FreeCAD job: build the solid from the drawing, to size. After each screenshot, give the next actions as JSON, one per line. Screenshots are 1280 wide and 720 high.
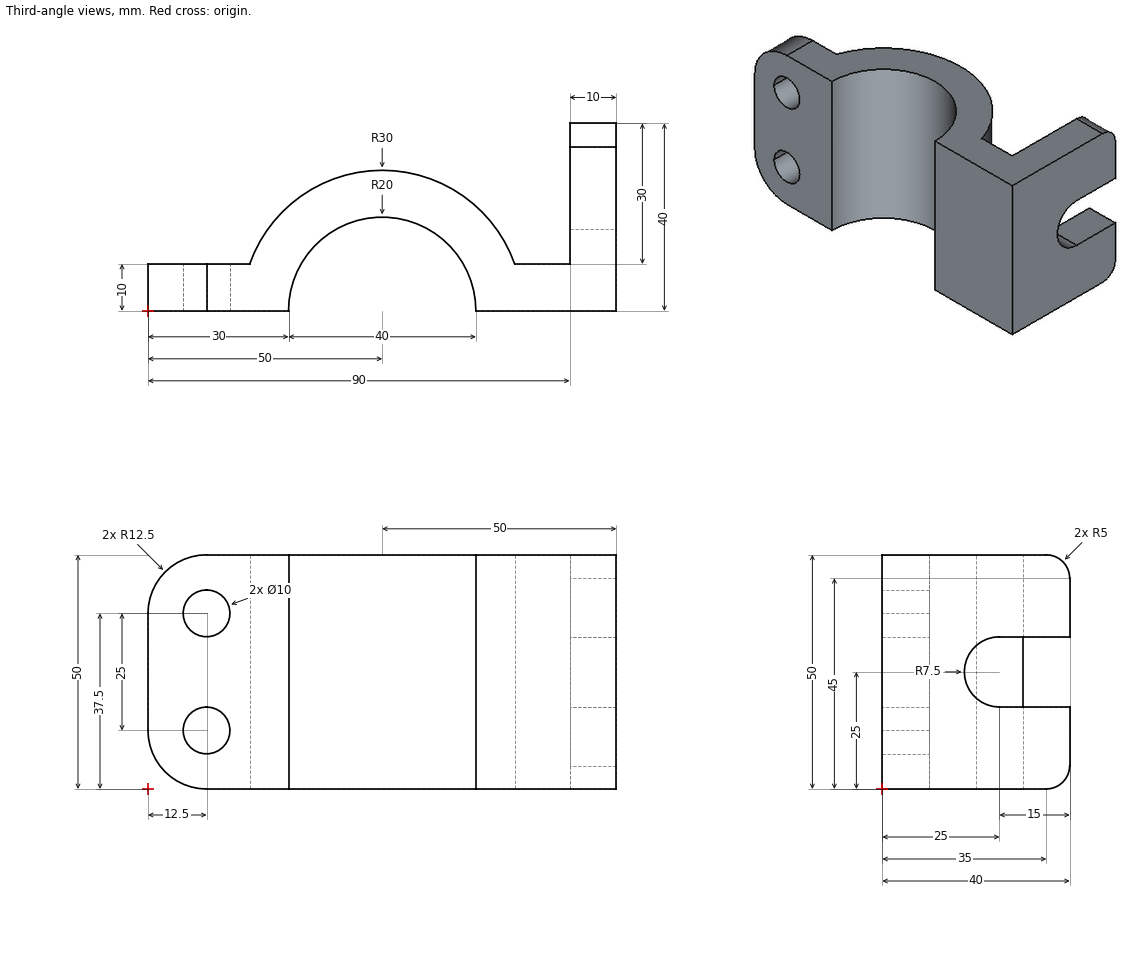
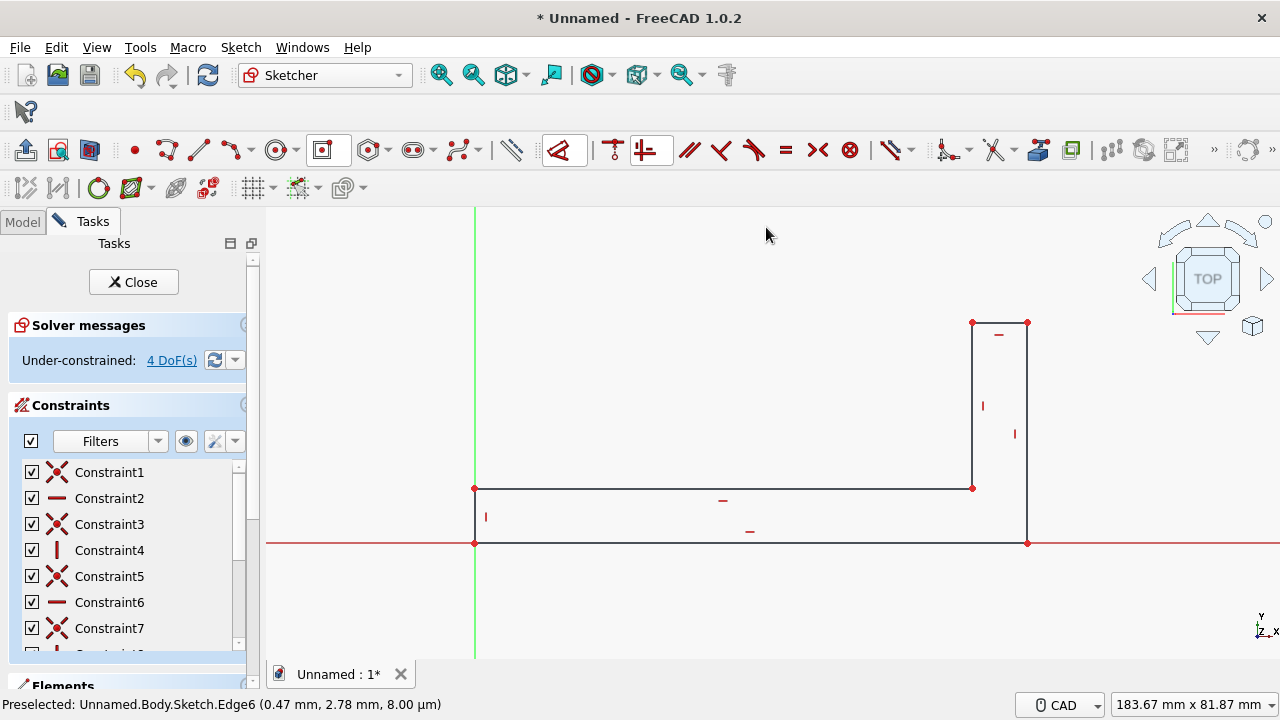
{"action": "left_click", "coordinate": [558, 150]}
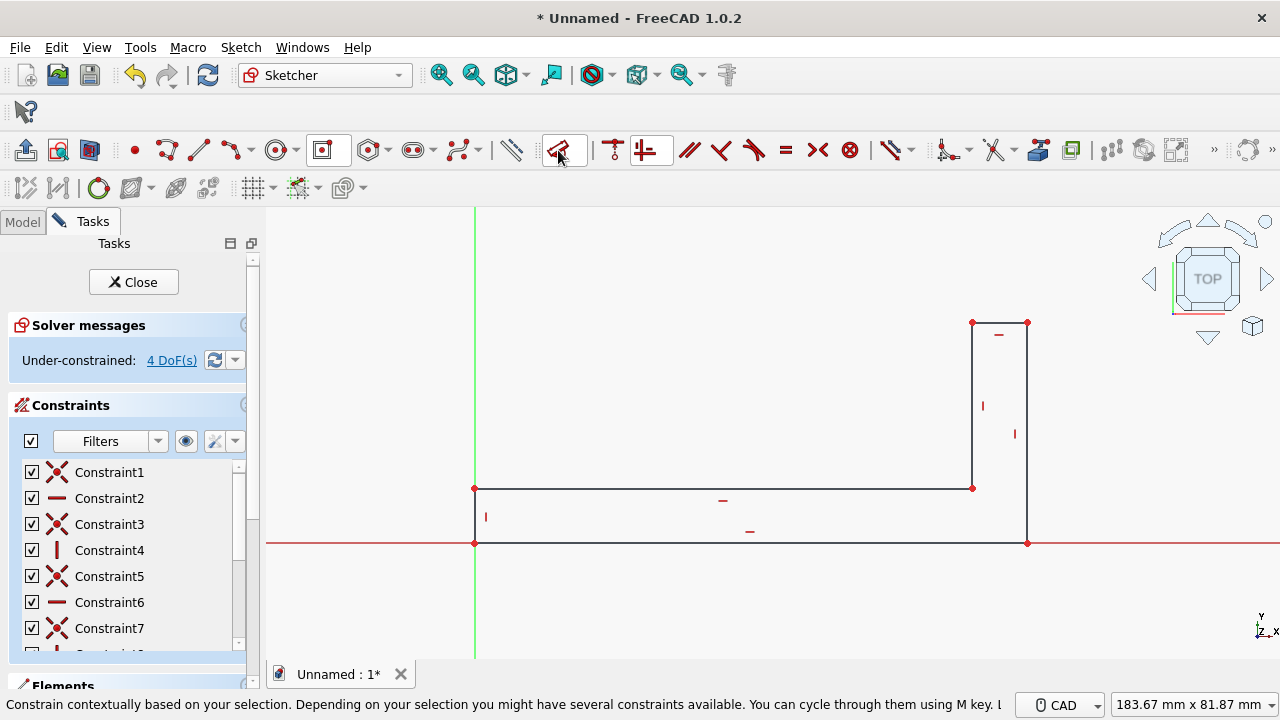
{"action": "left_click", "coordinate": [1027, 477]}
{"action": "left_click", "coordinate": [1061, 433]}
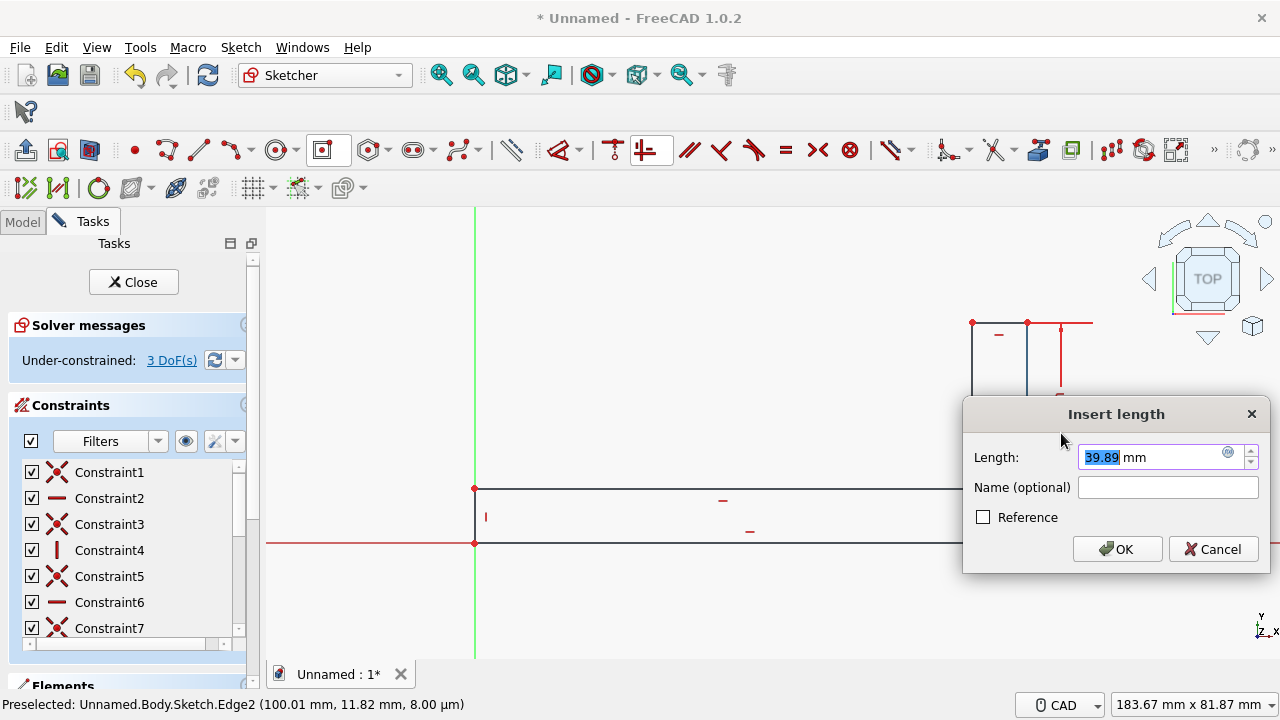
{"action": "type", "text": "40"}
{"action": "key", "text": "Return"}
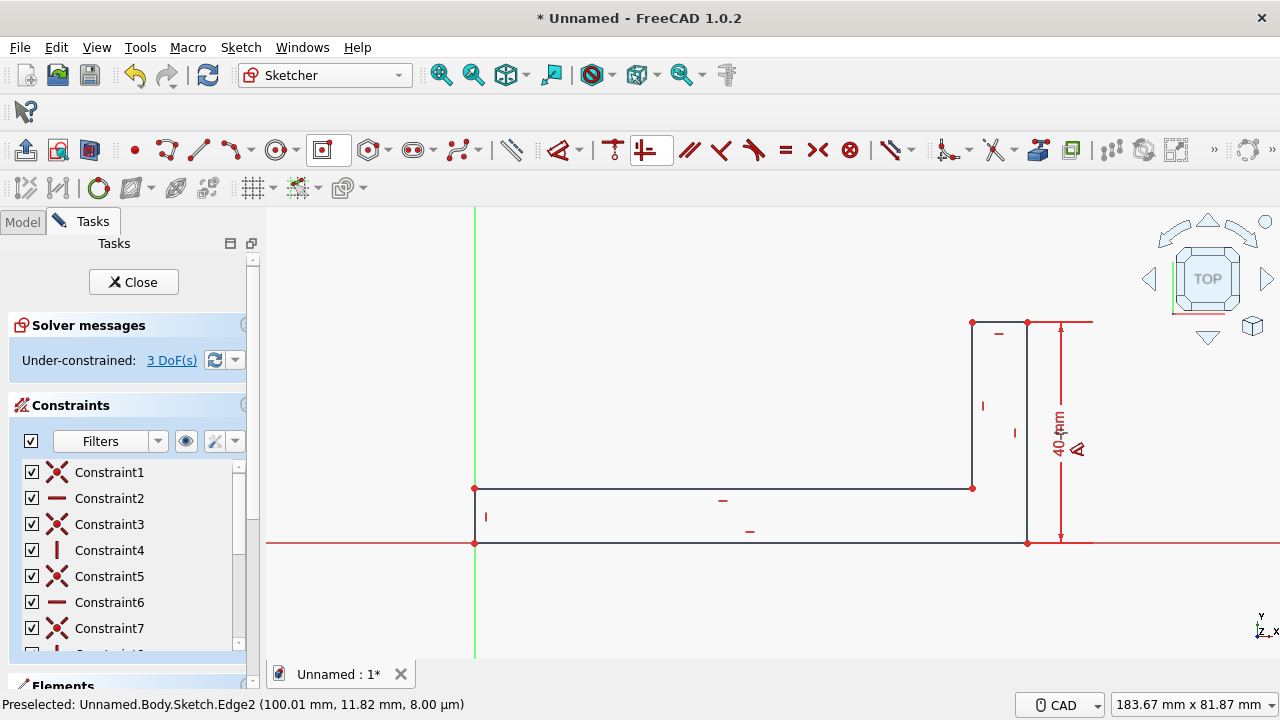
{"action": "left_click", "coordinate": [1010, 322]}
{"action": "left_click", "coordinate": [999, 288]}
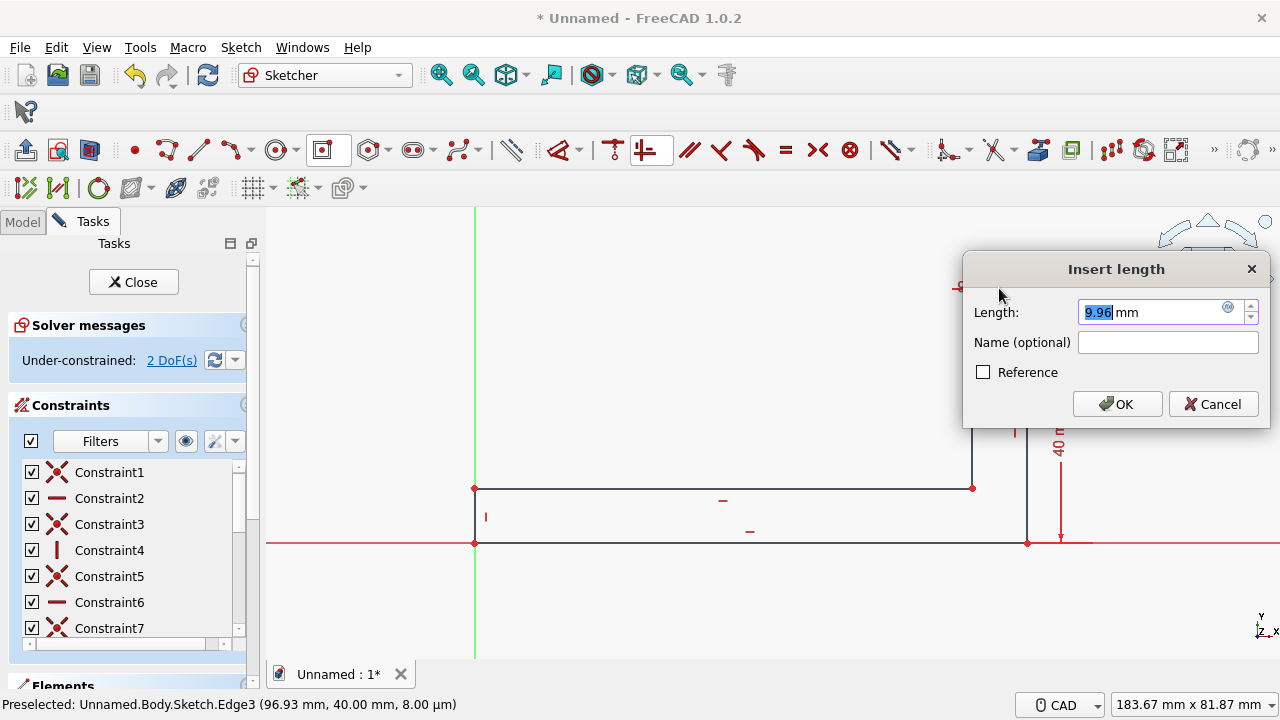
{"action": "type", "text": "10"}
{"action": "key", "text": "Return"}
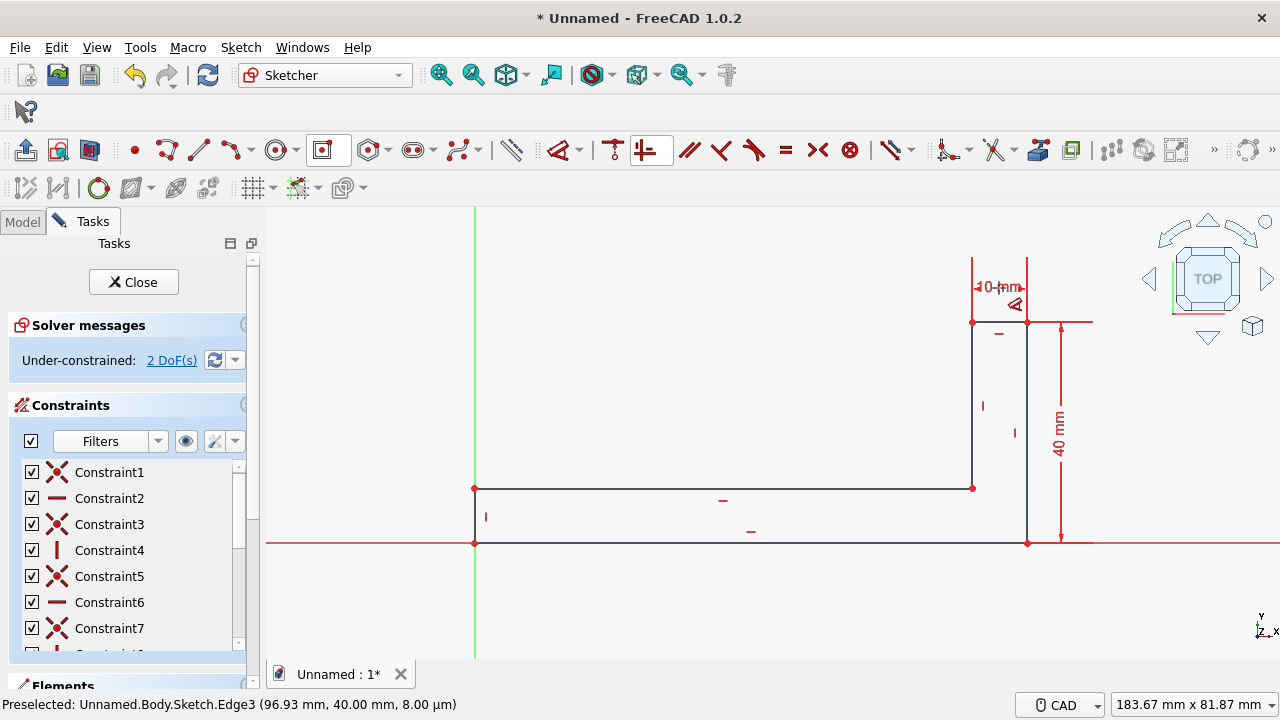
{"action": "left_click", "coordinate": [972, 372]}
{"action": "left_click", "coordinate": [1006, 406]}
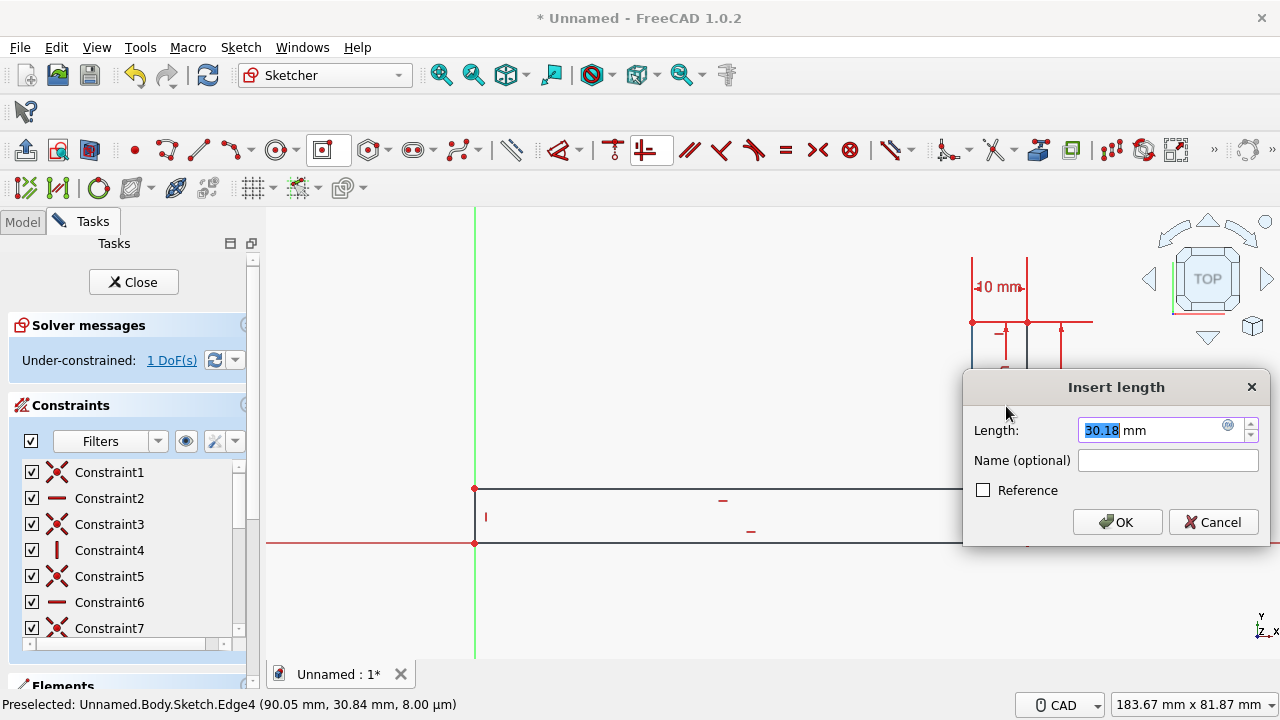
{"action": "type", "text": "30"}
{"action": "key", "text": "Return"}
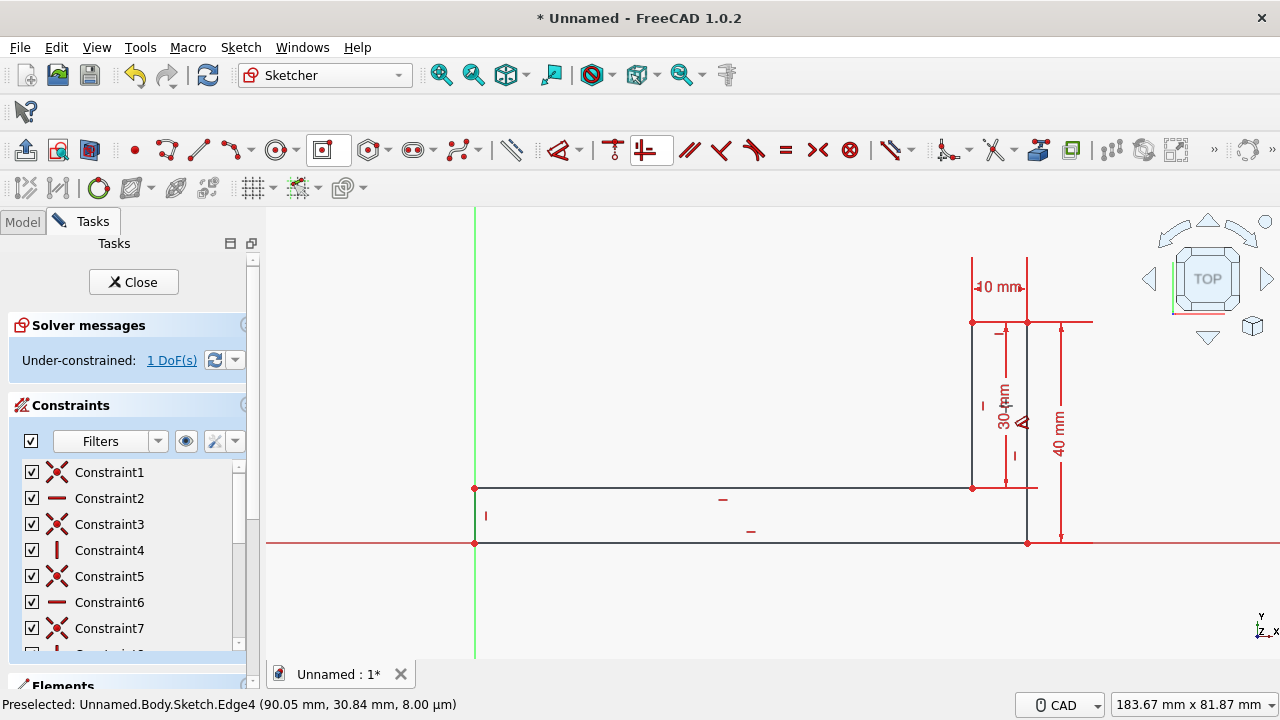
{"action": "left_click", "coordinate": [823, 488]}
{"action": "left_click", "coordinate": [723, 522]}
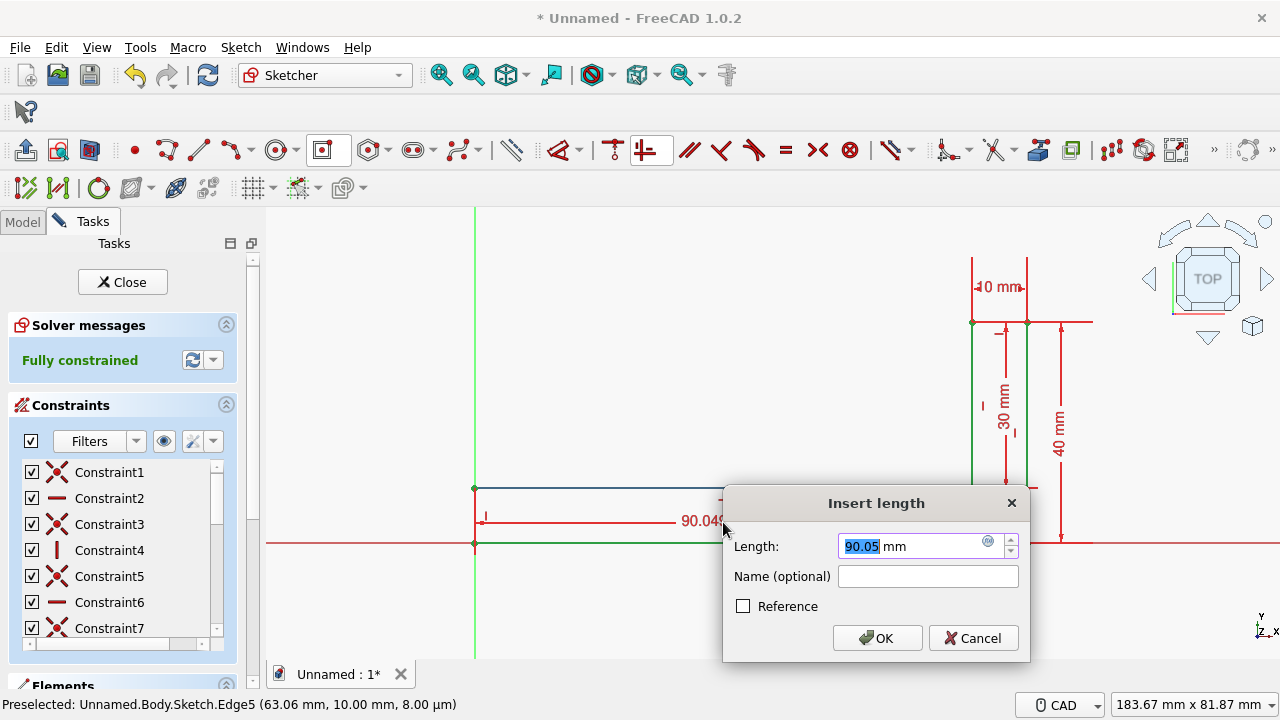
{"action": "type", "text": "90"}
{"action": "key", "text": "Return"}
{"action": "key", "text": "Escape"}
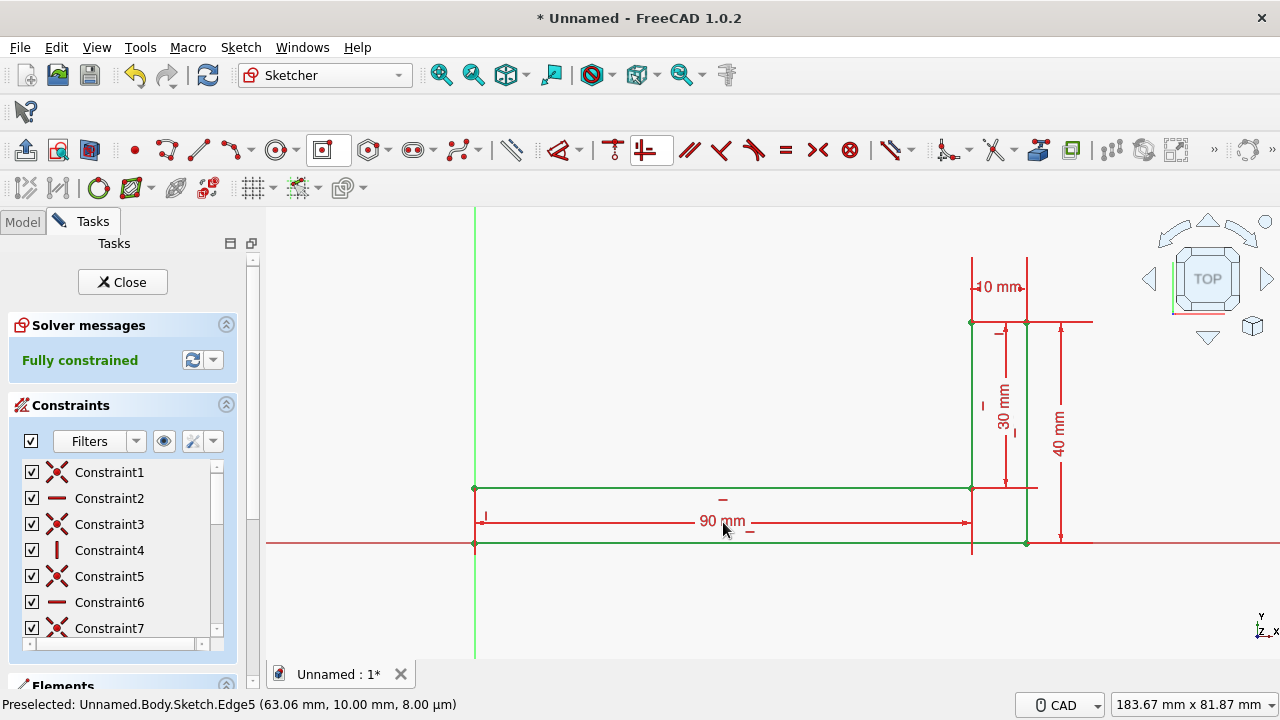
{"action": "left_click", "coordinate": [123, 282]}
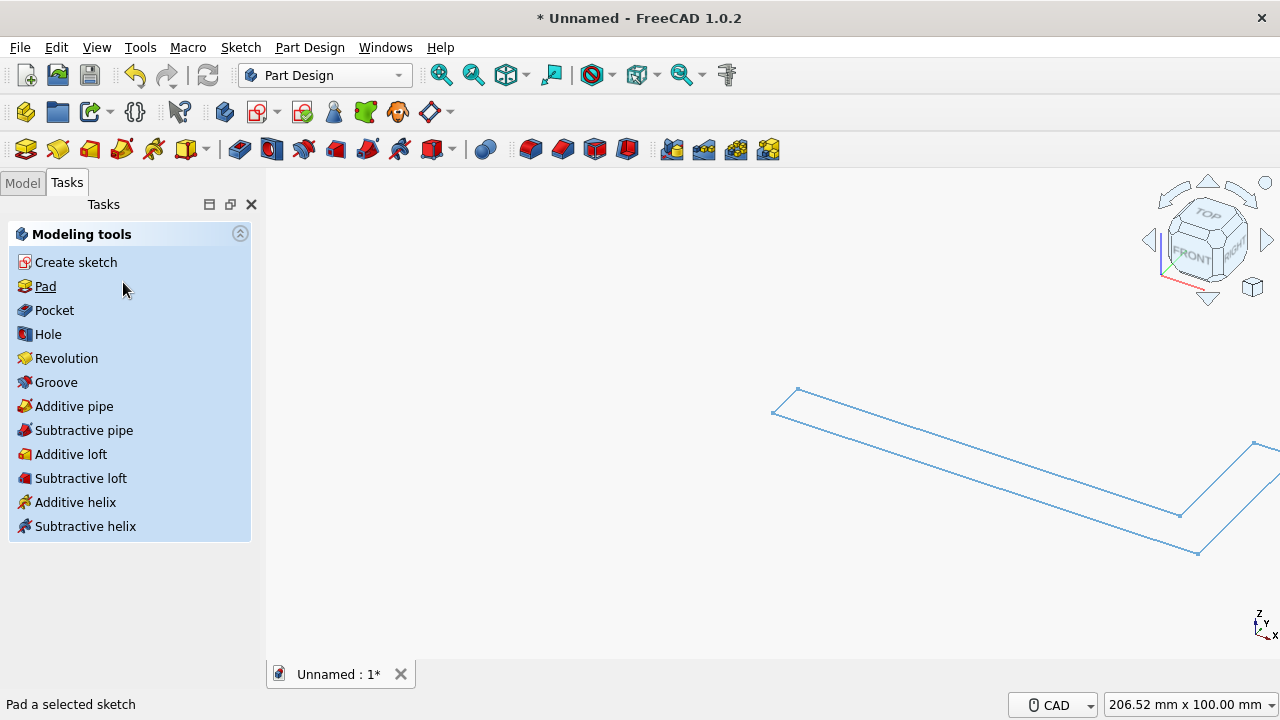
{"action": "left_click", "coordinate": [26, 150]}